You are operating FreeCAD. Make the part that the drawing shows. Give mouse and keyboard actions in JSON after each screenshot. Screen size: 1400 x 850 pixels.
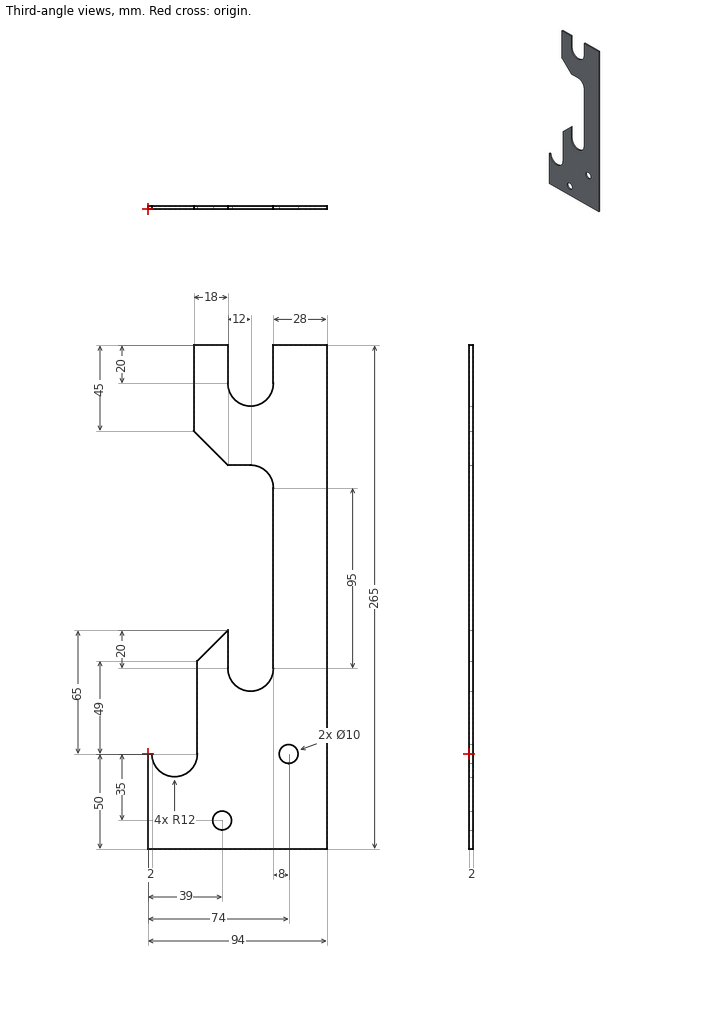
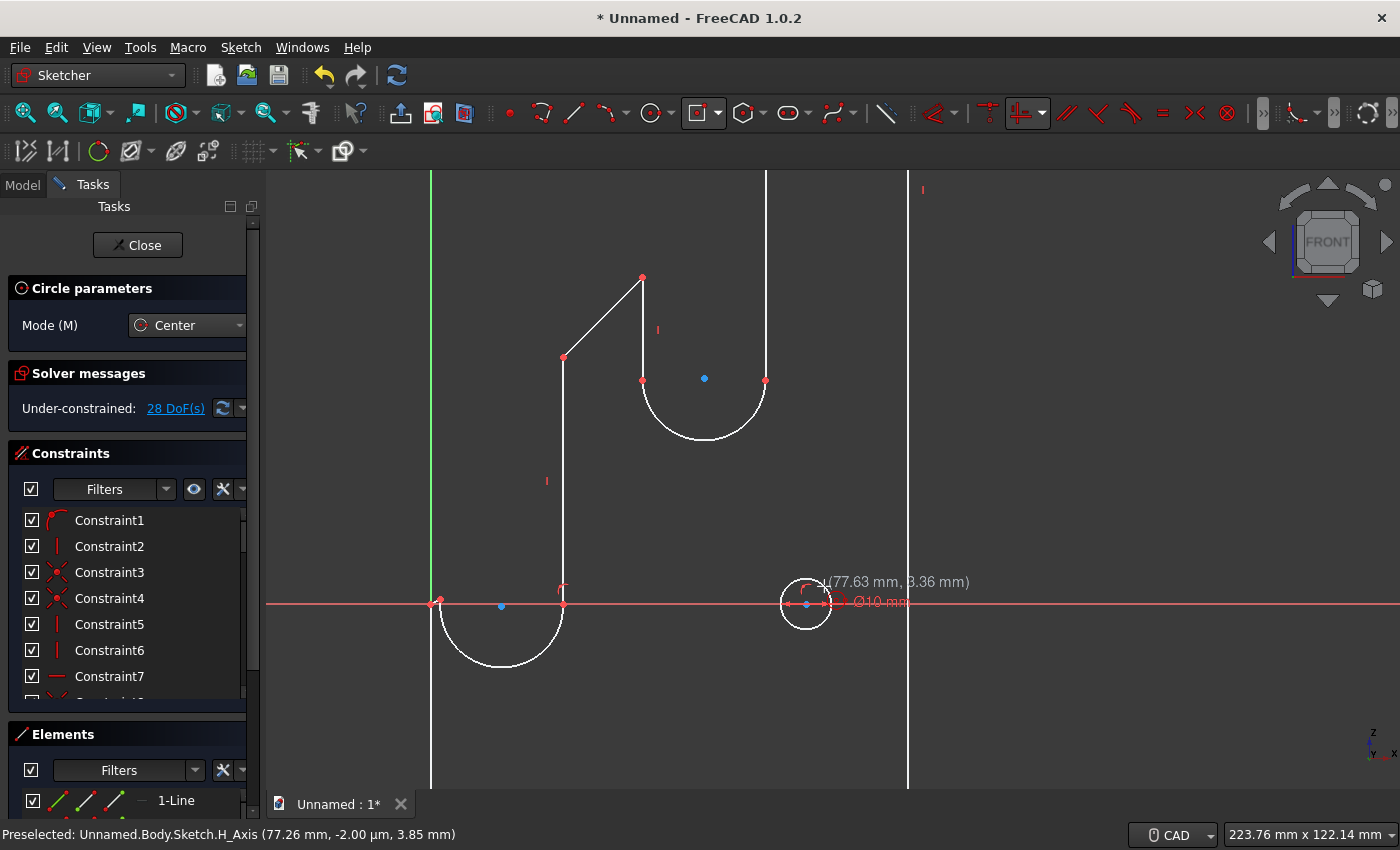
{"action": "scroll", "coordinate": [806, 606], "scroll_direction": "down", "scroll_amount": 6}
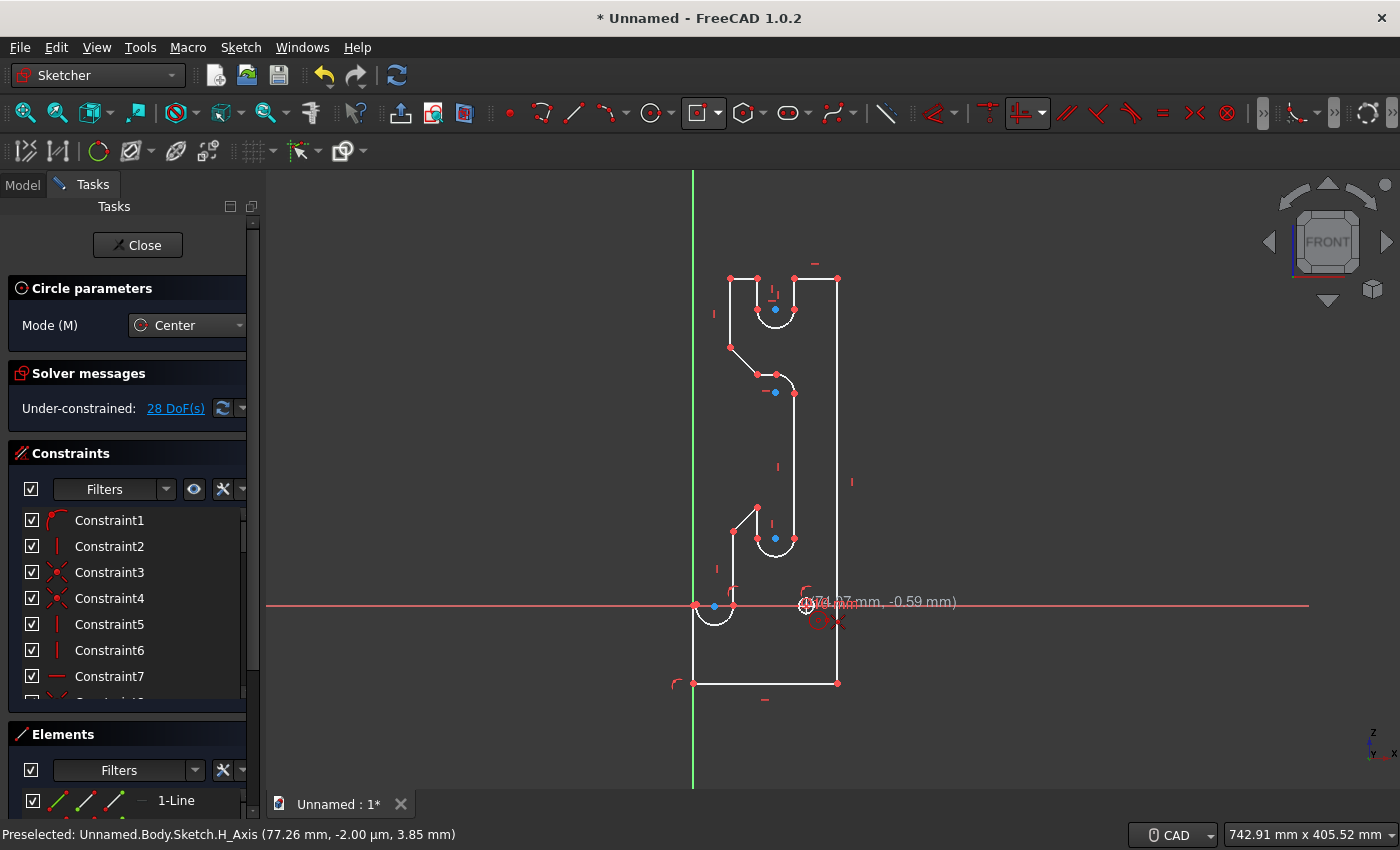
{"action": "scroll", "coordinate": [753, 659], "scroll_direction": "up", "scroll_amount": 6}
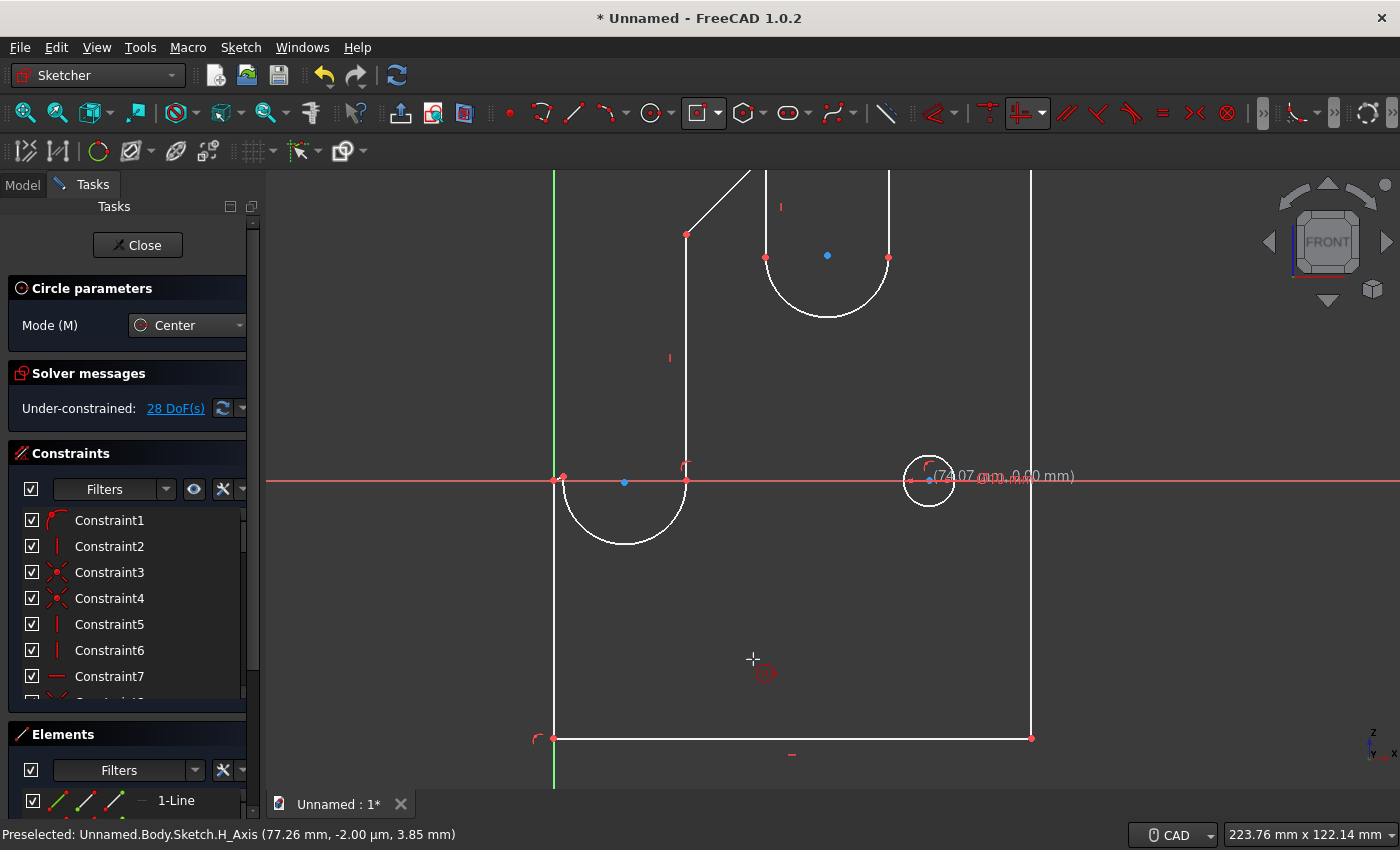
{"action": "left_click", "coordinate": [751, 658]}
{"action": "mouse_move", "coordinate": [769, 640]}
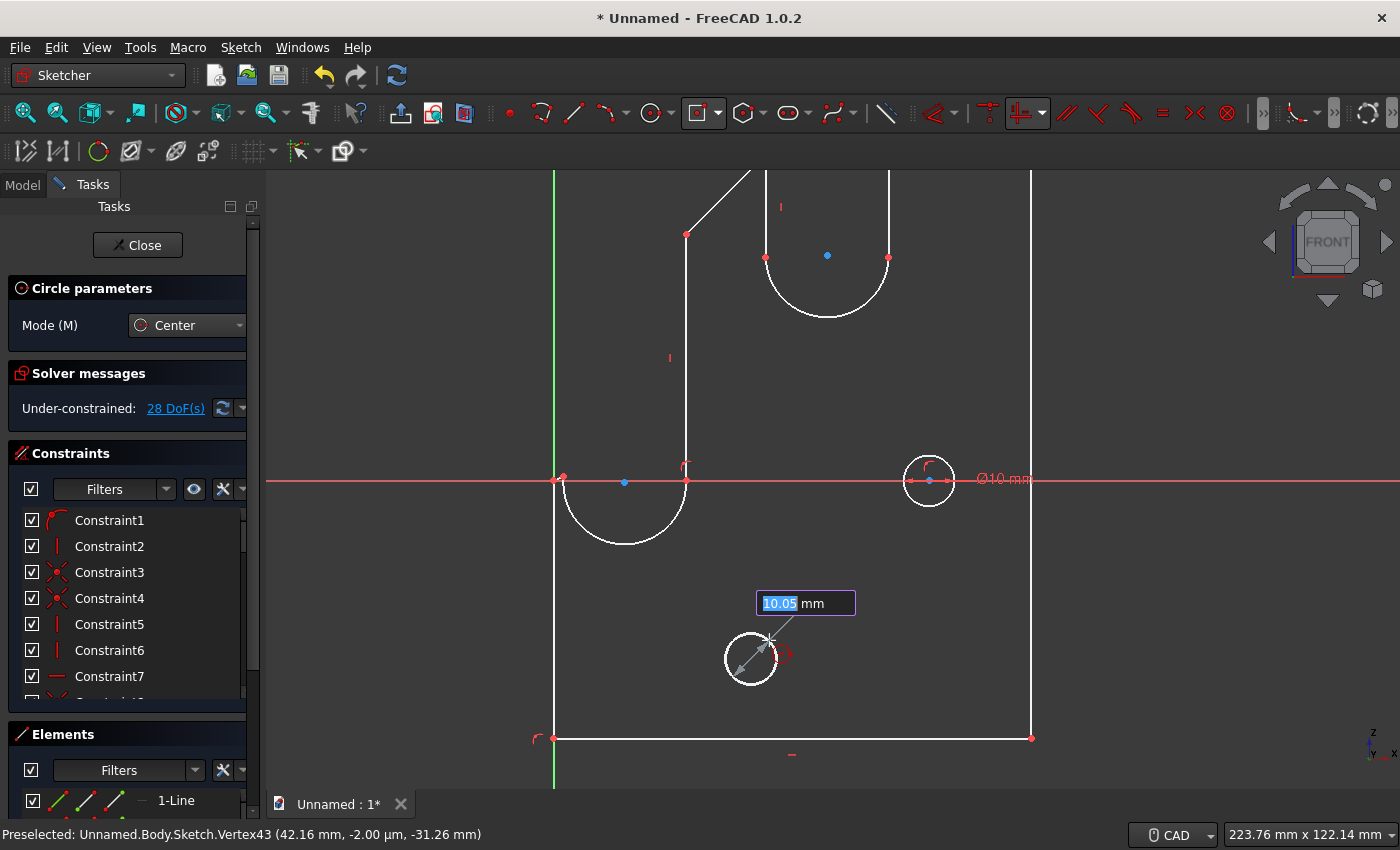
{"action": "type", "text": "10"}
{"action": "key", "text": "Return"}
{"action": "key", "text": "Escape"}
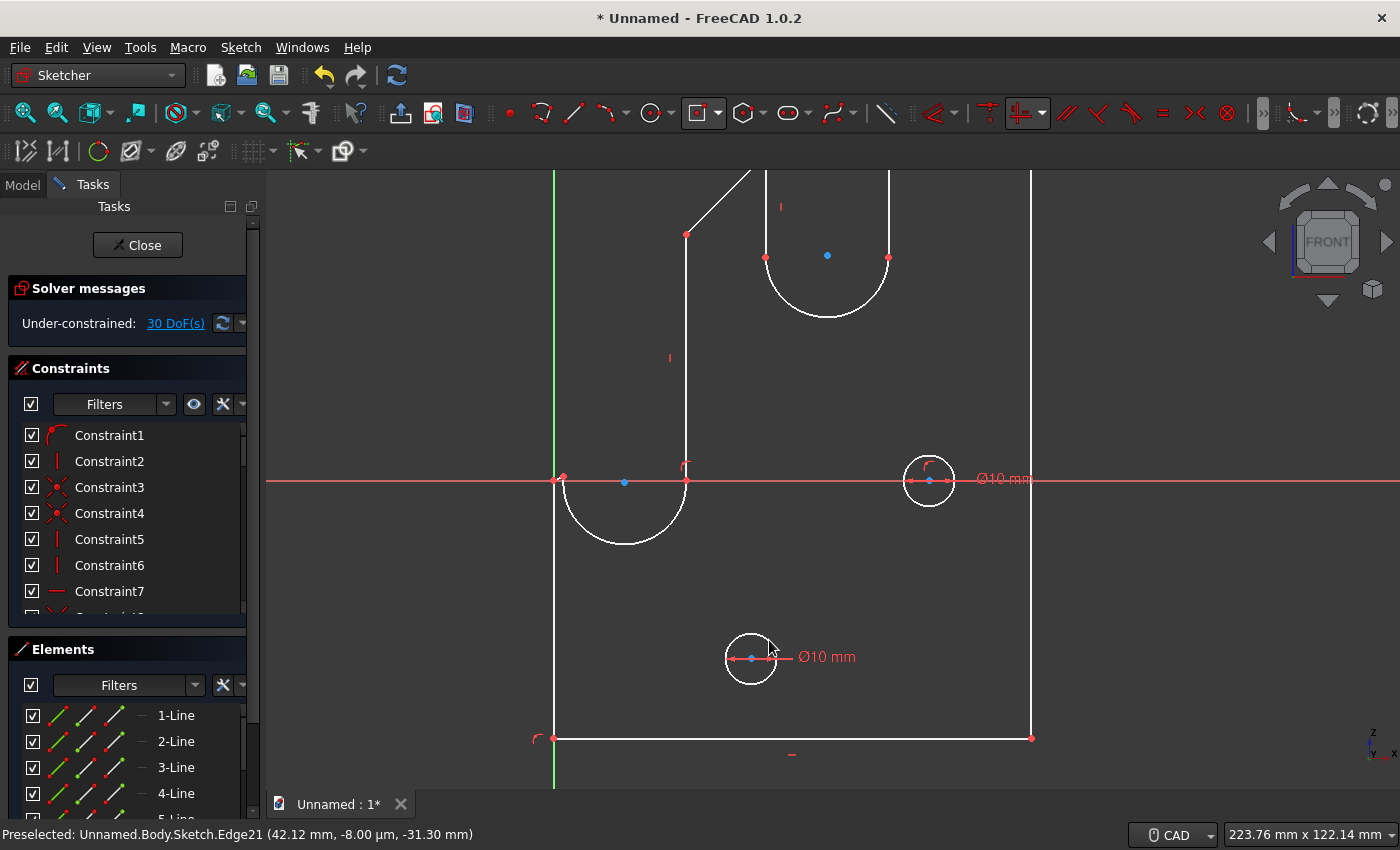
{"action": "left_click", "coordinate": [686, 407]}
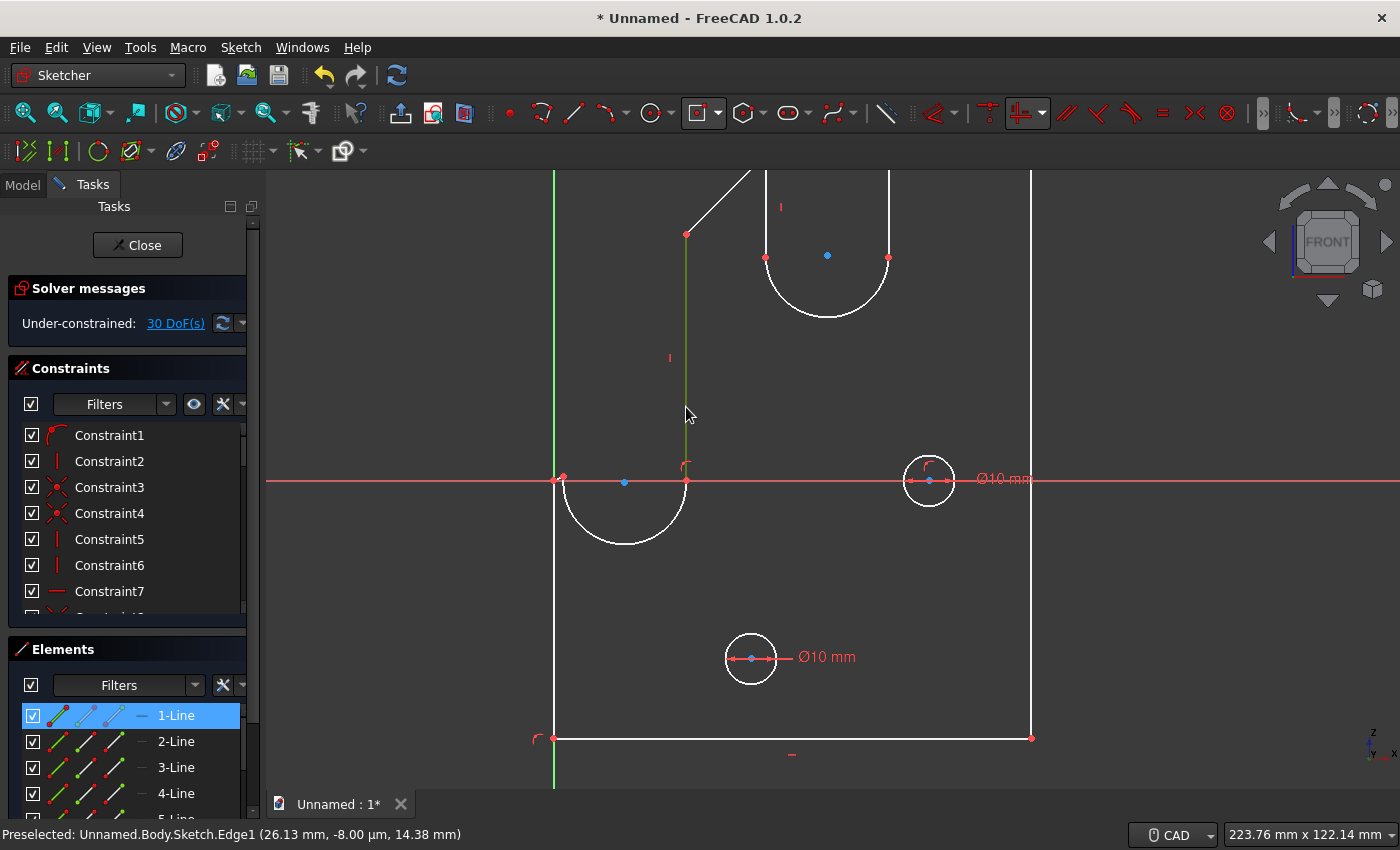
{"action": "left_click", "coordinate": [586, 530]}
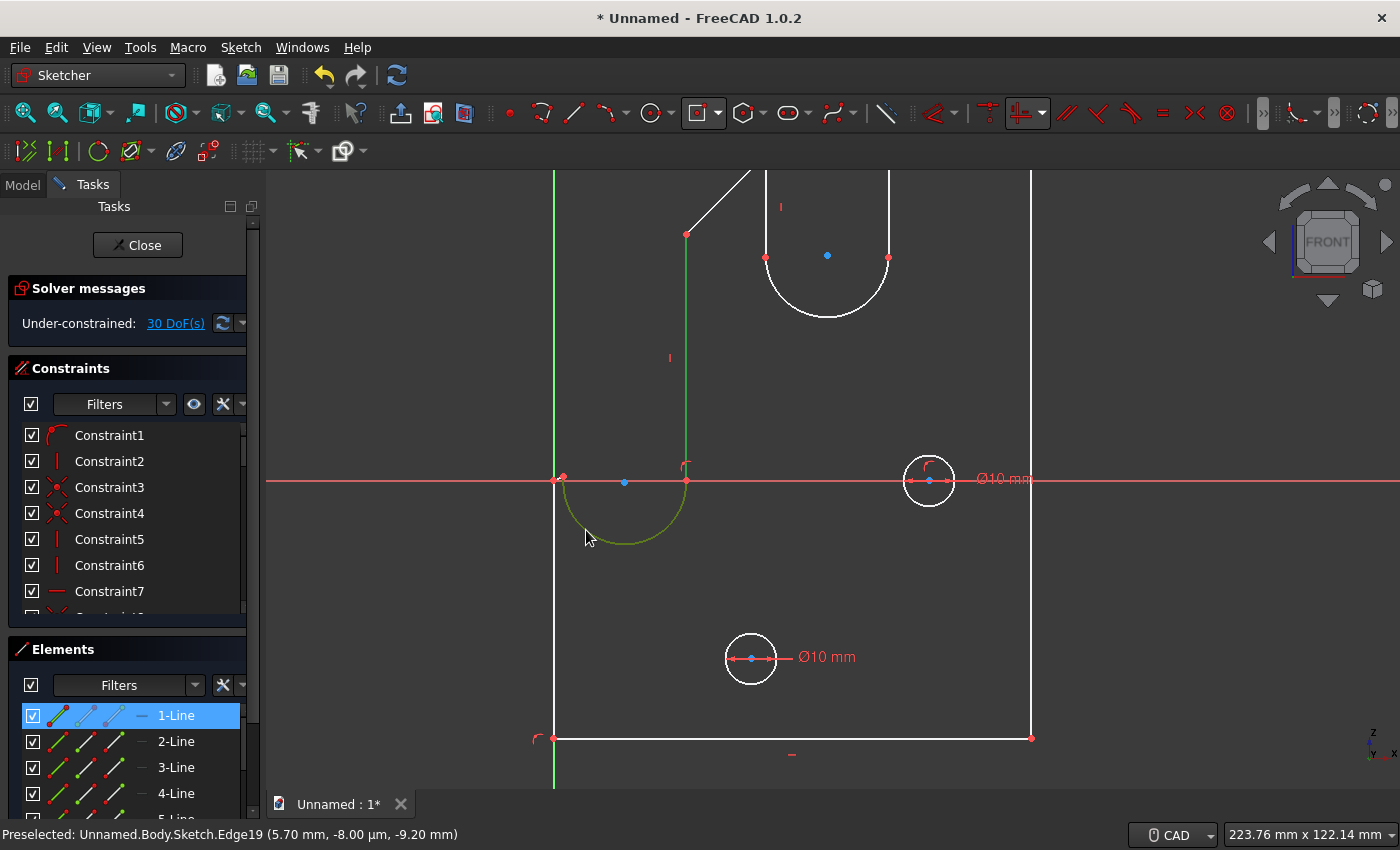
{"action": "left_click", "coordinate": [1132, 114]}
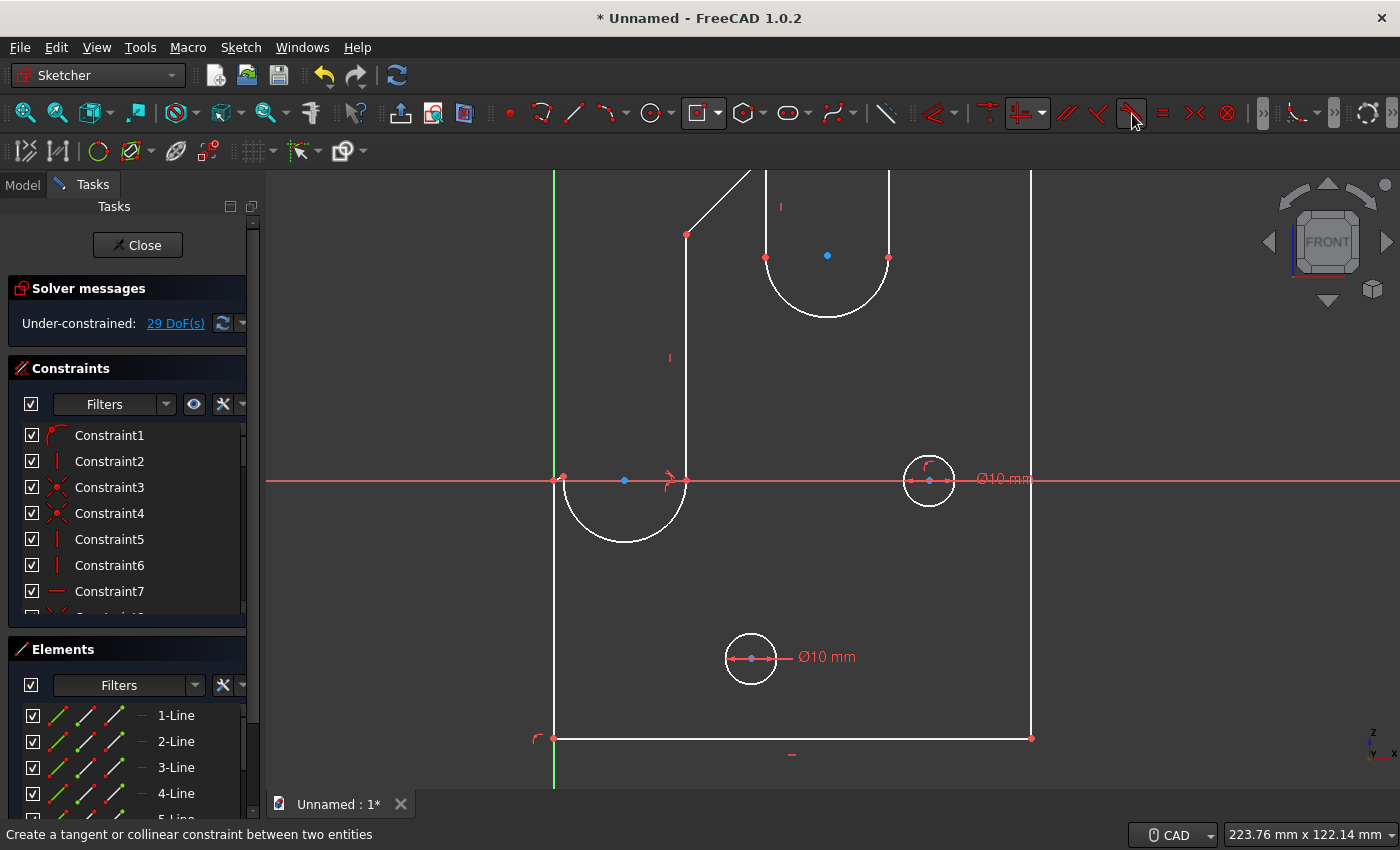
{"action": "left_click", "coordinate": [766, 227]}